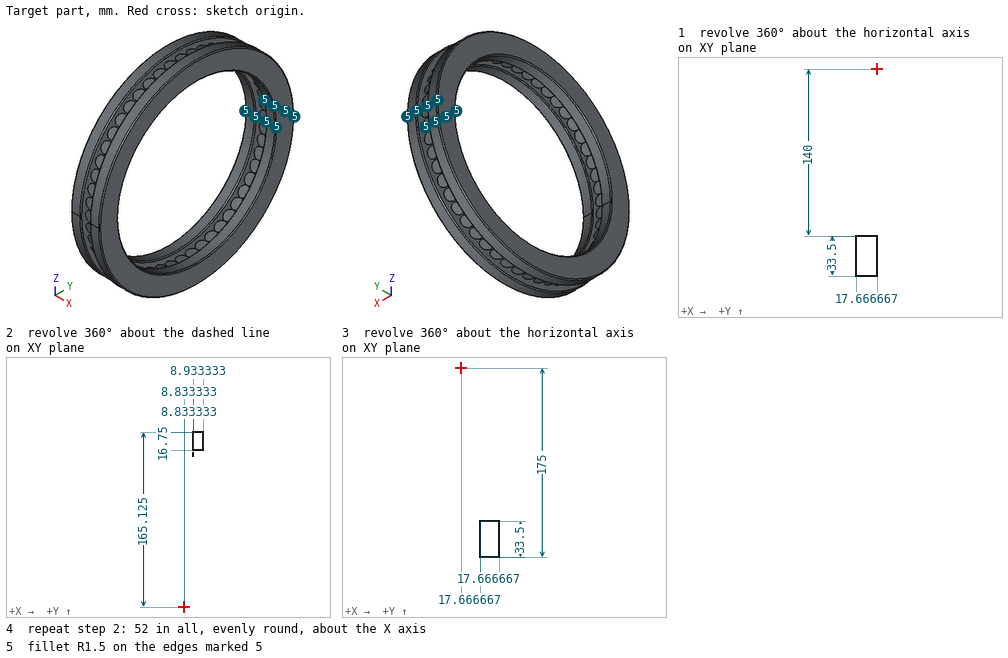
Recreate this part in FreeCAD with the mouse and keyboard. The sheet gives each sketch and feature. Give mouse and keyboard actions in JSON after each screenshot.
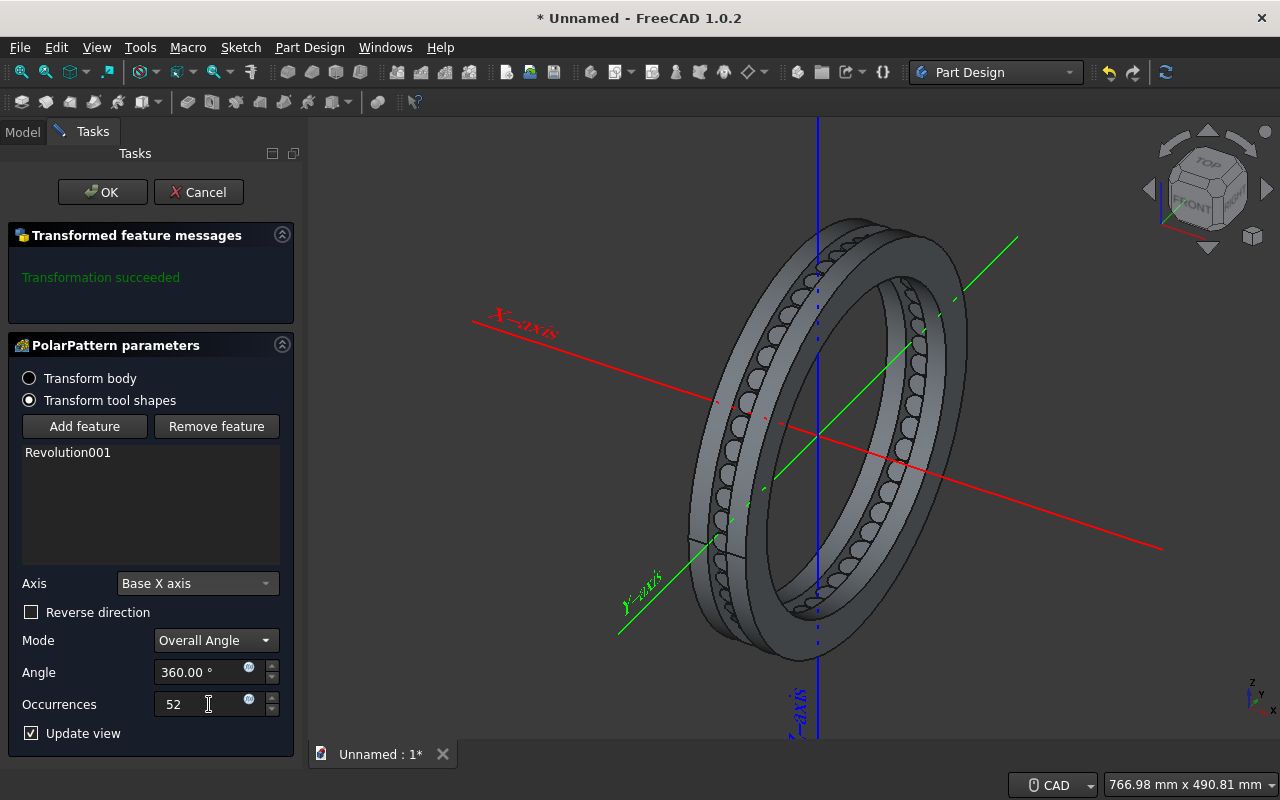
{"action": "left_click", "coordinate": [103, 192]}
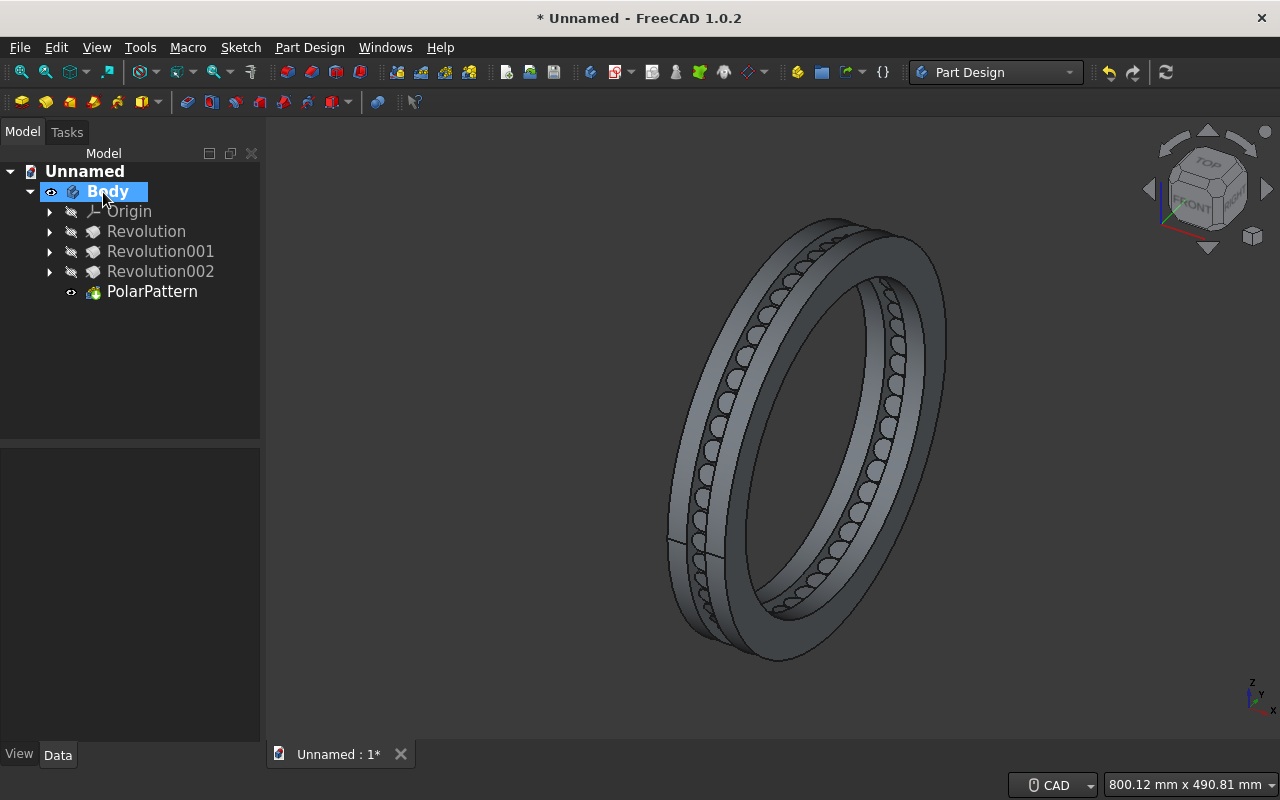
{"action": "left_click", "coordinate": [870, 241]}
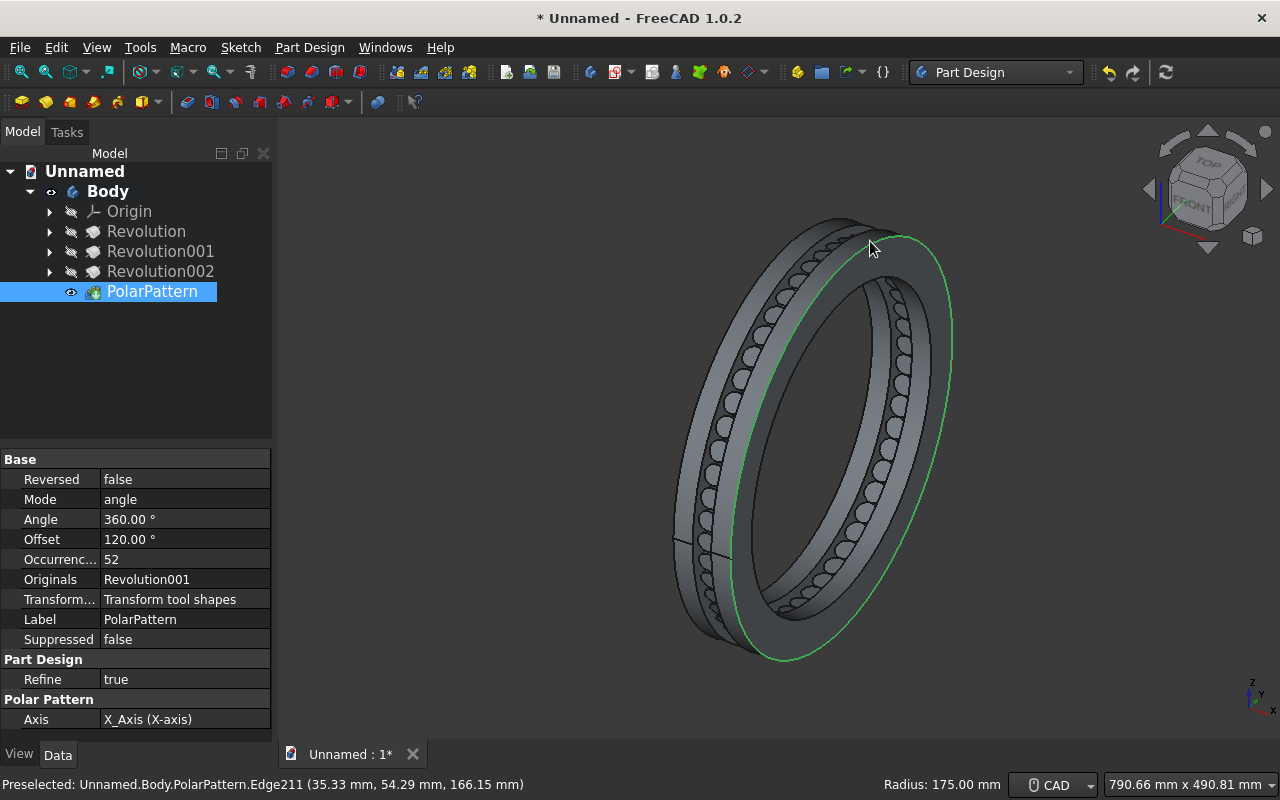
{"action": "left_click", "coordinate": [931, 358], "text": "ctrl"}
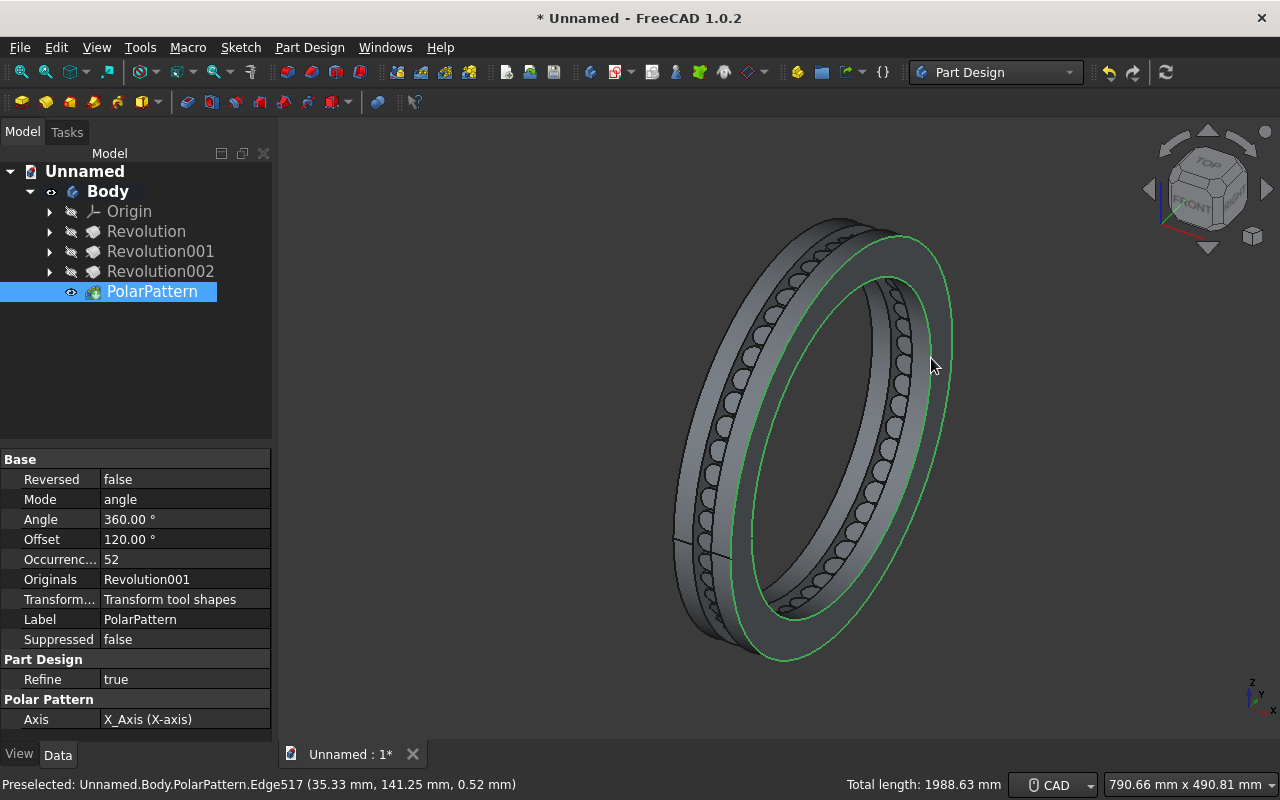
{"action": "left_click", "coordinate": [837, 230], "text": "ctrl"}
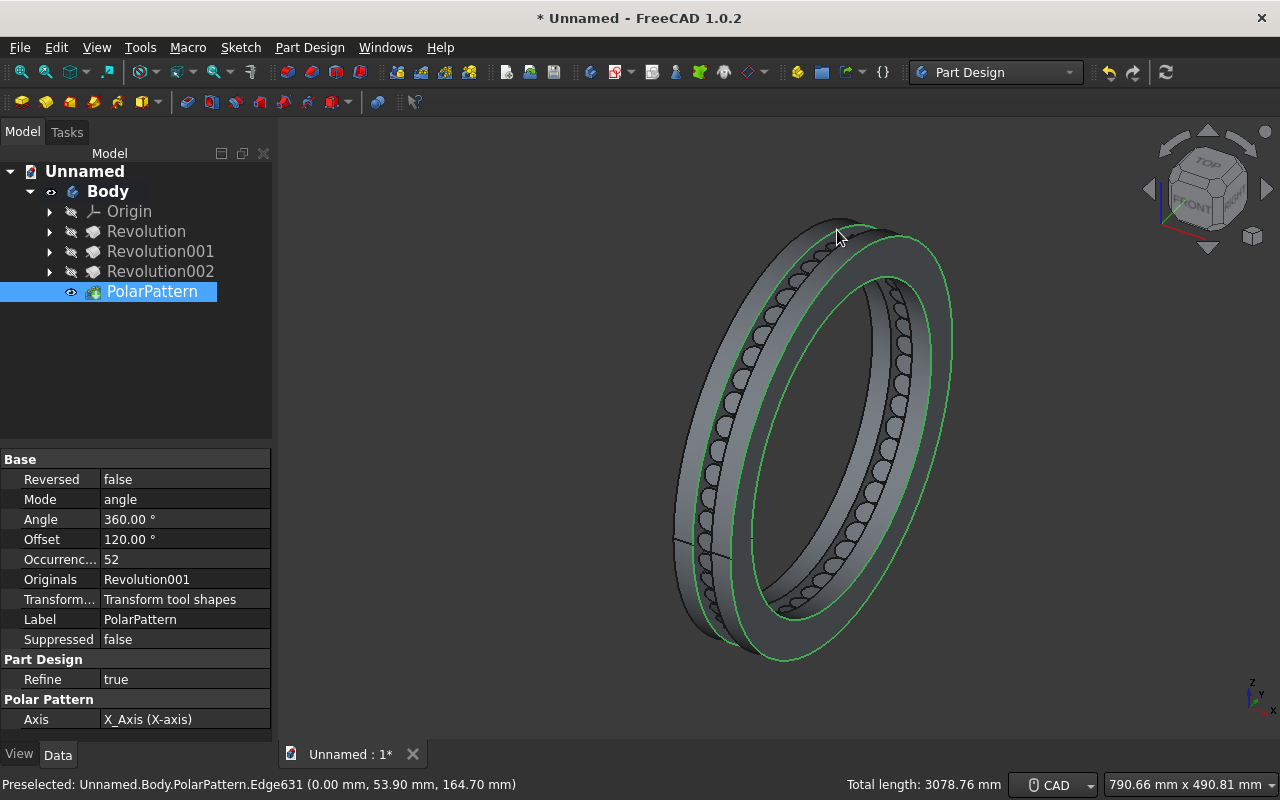
{"action": "left_click", "coordinate": [891, 346], "text": "ctrl"}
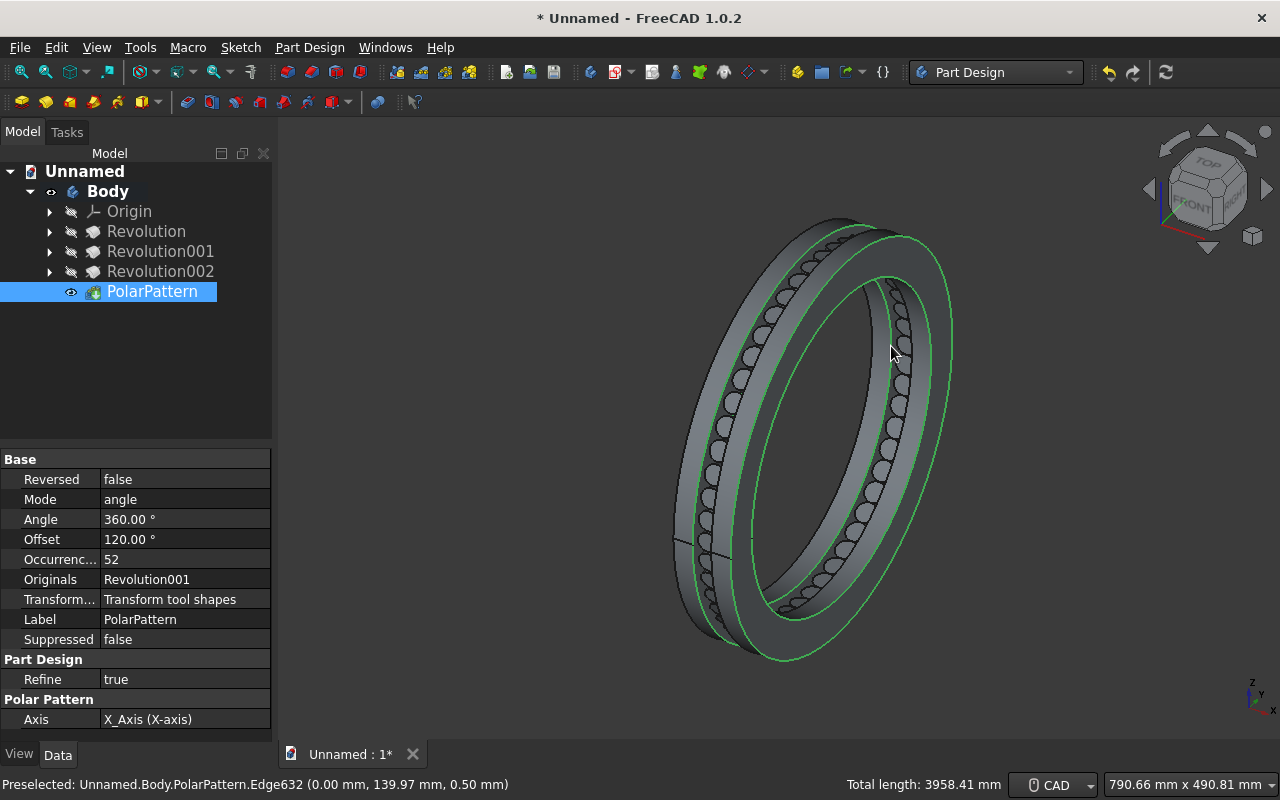
{"action": "key", "text": "0"}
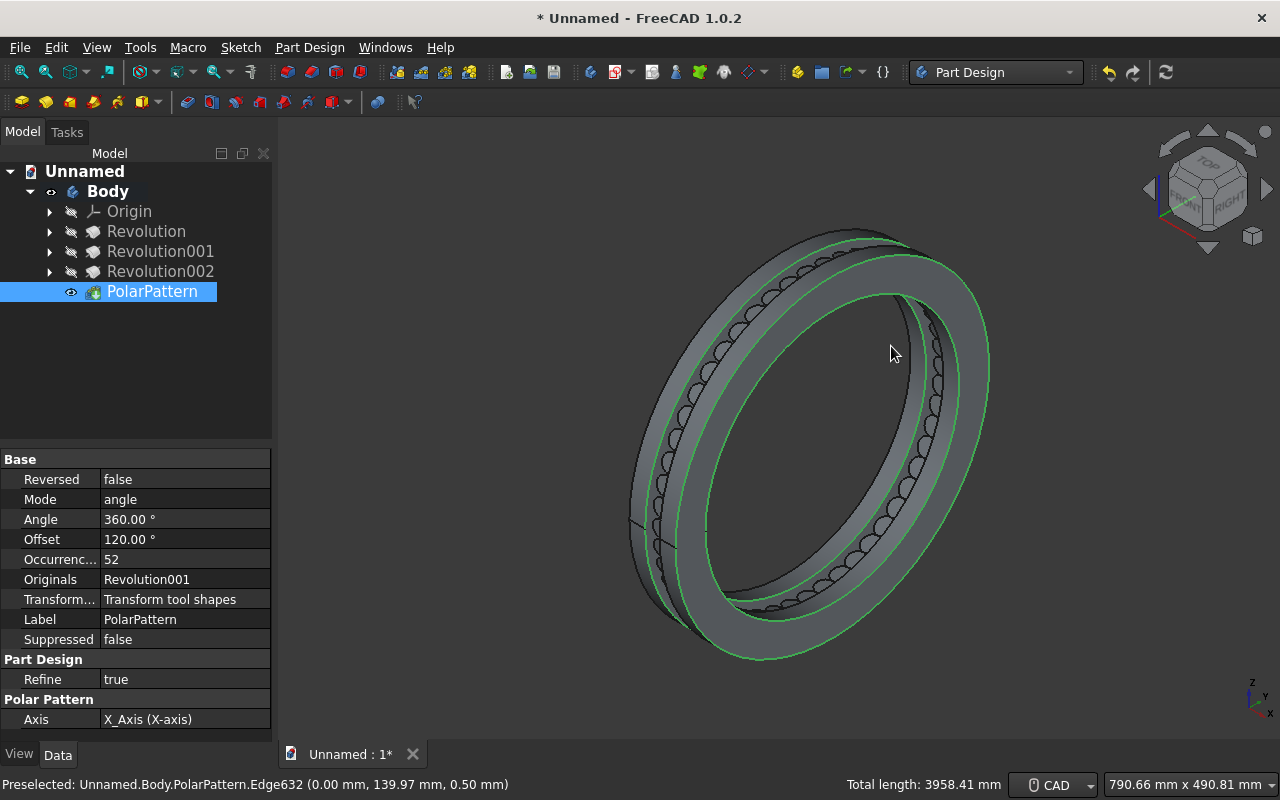
{"action": "left_click", "coordinate": [737, 286], "text": "ctrl"}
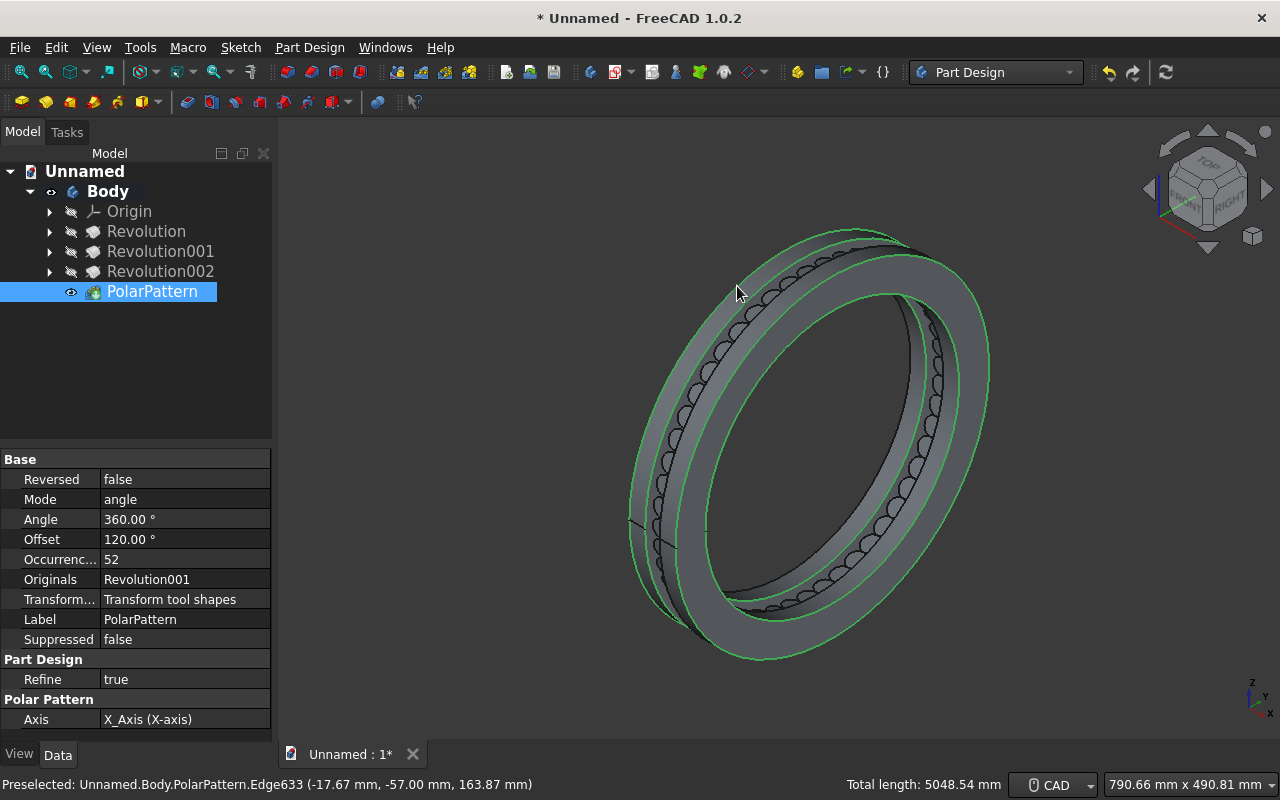
{"action": "key", "text": "2"}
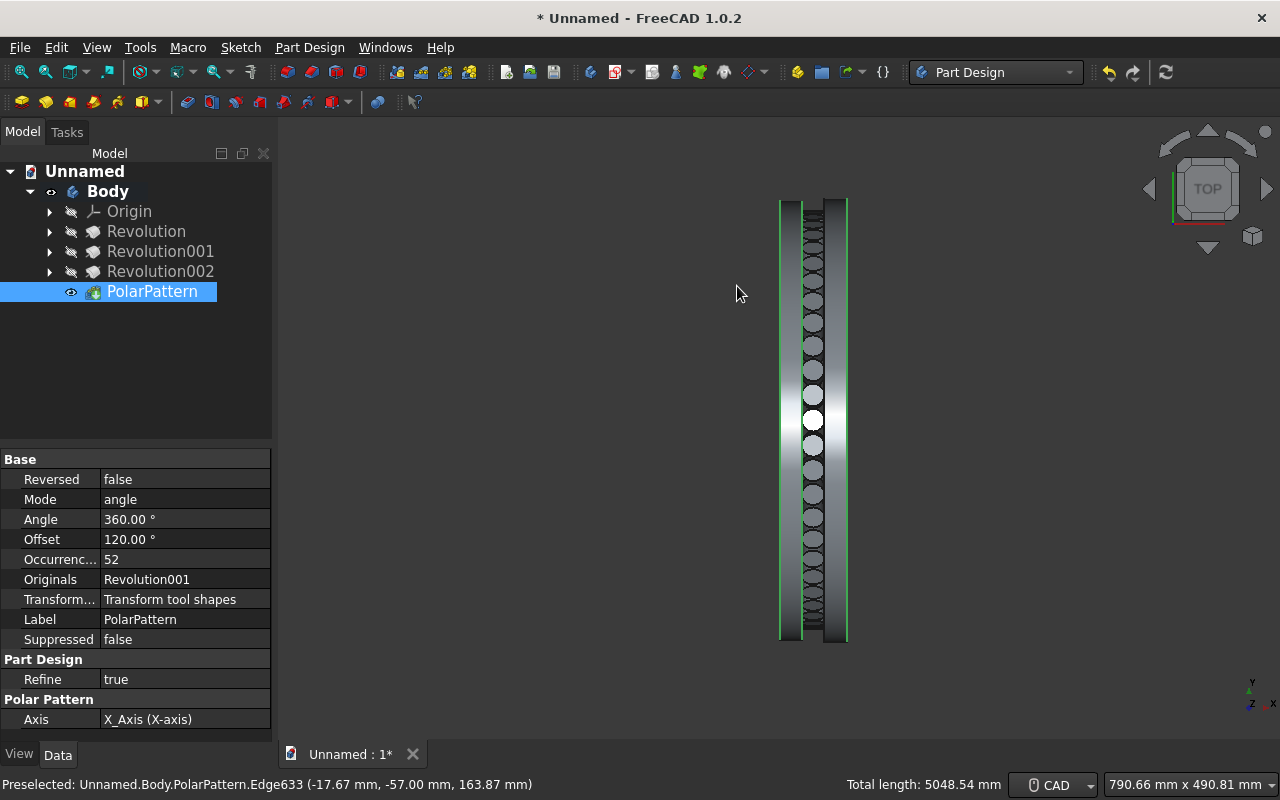
{"action": "left_click", "coordinate": [824, 240], "text": "ctrl"}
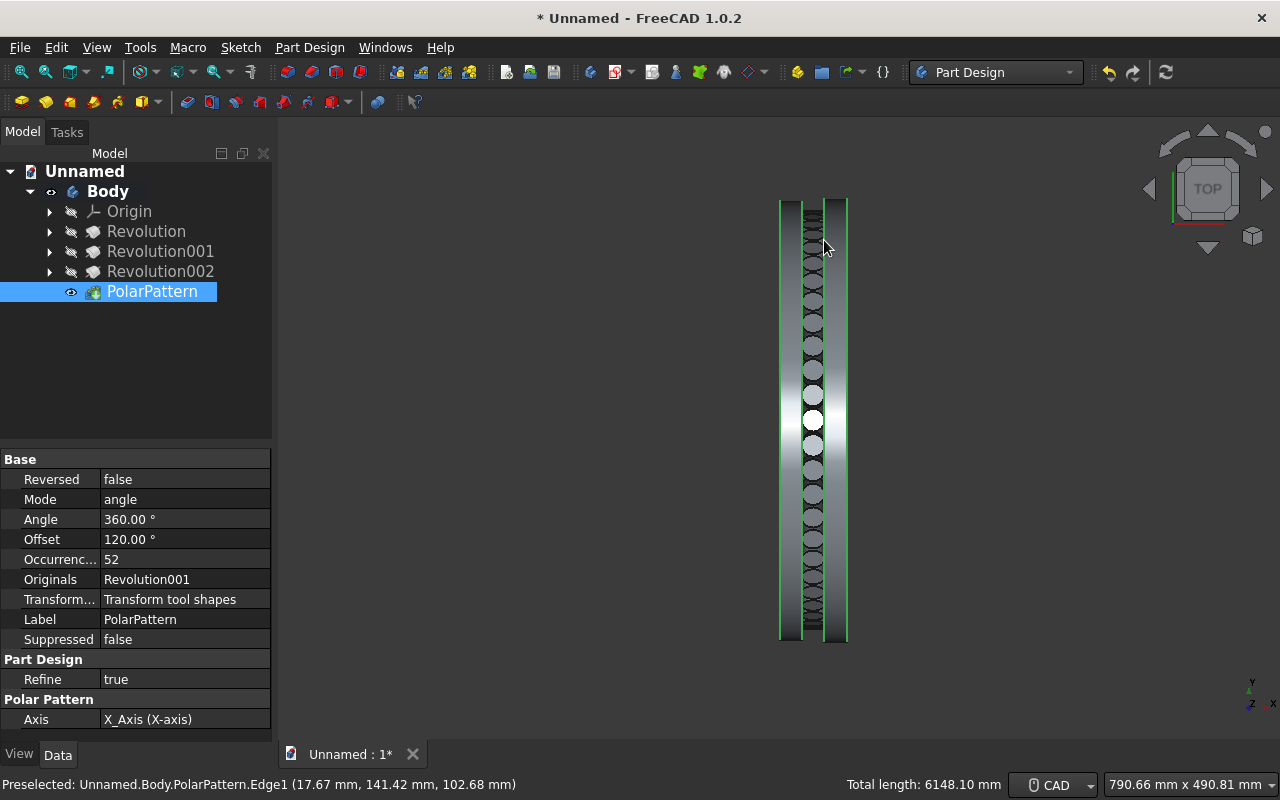
{"action": "key", "text": "1"}